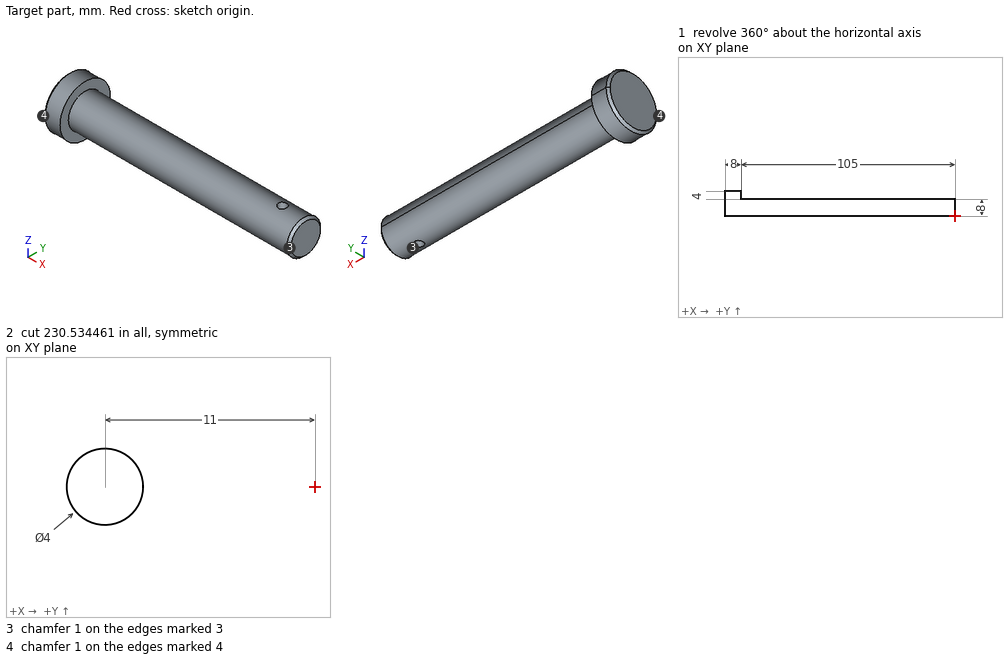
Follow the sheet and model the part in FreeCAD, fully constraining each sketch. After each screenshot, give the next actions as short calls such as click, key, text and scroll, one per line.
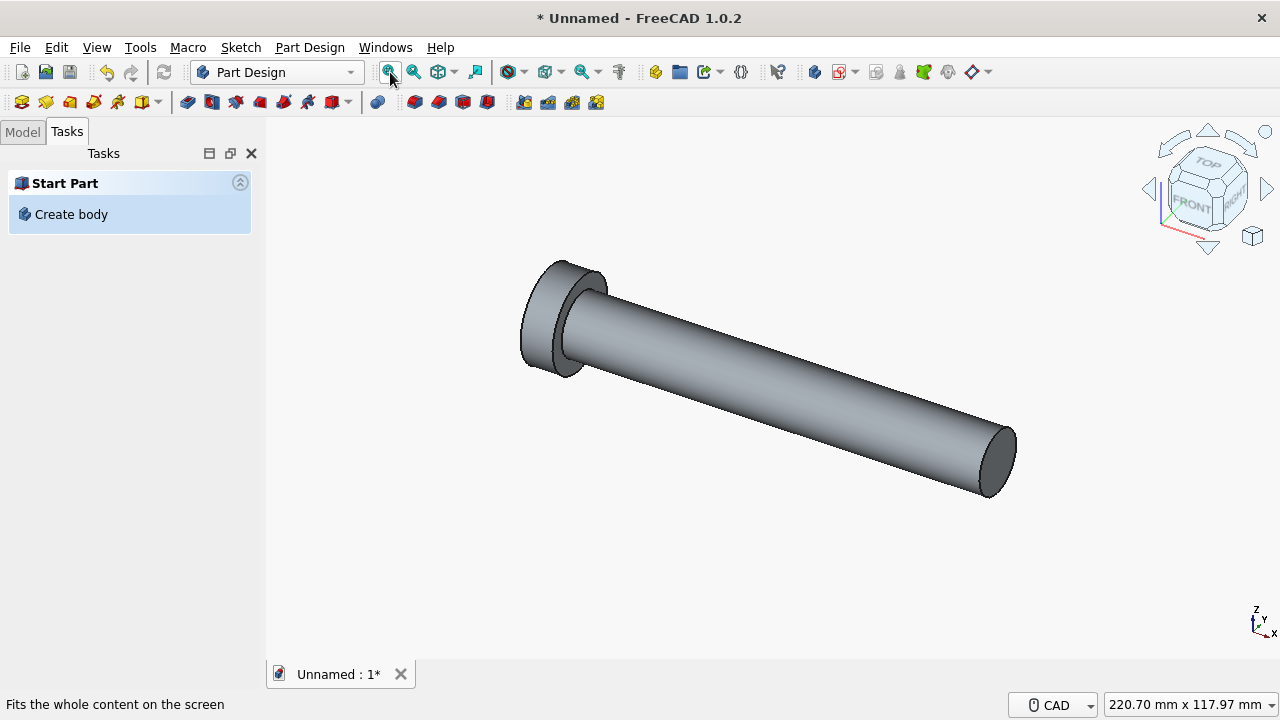
click(840, 72)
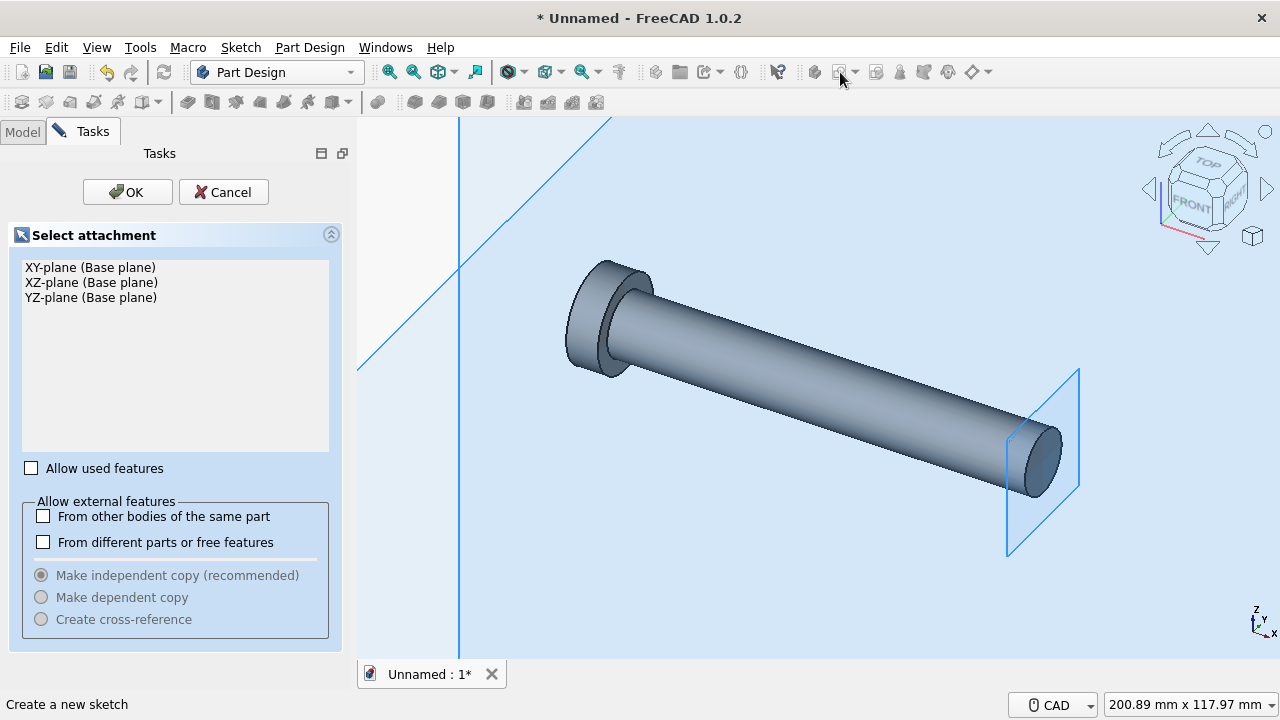
click(82, 268)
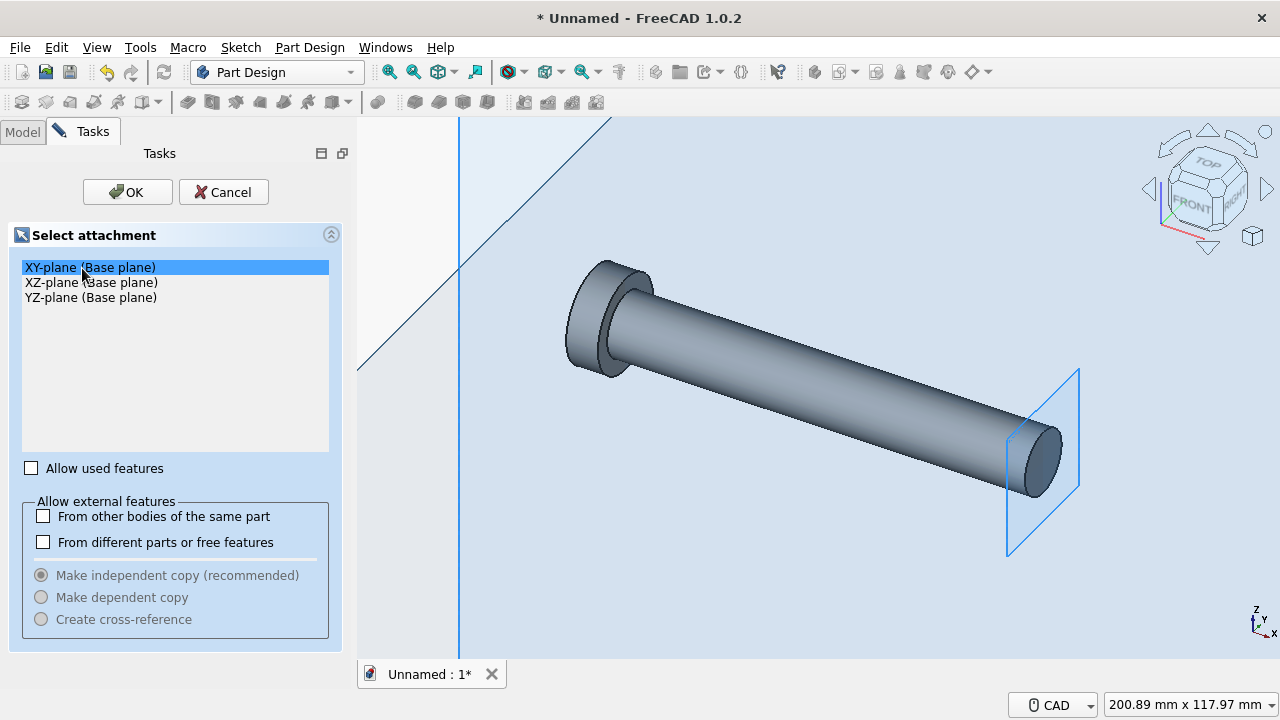
click(128, 192)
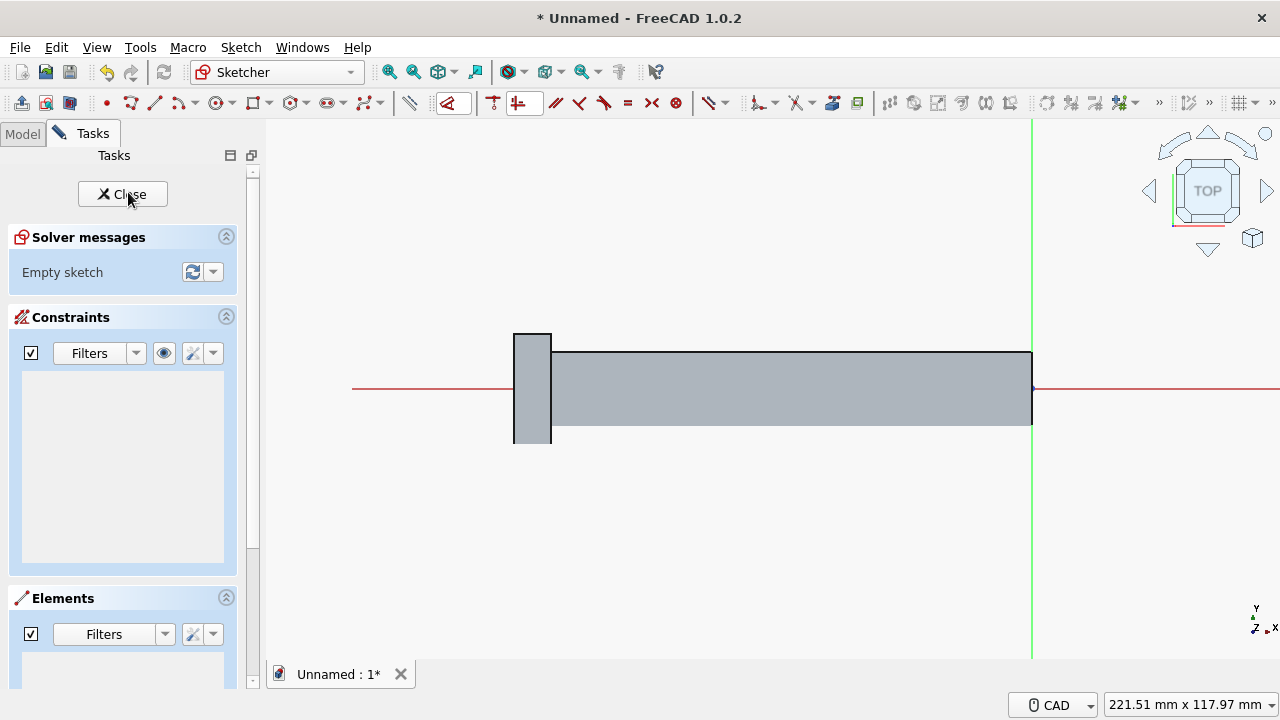
click(70, 104)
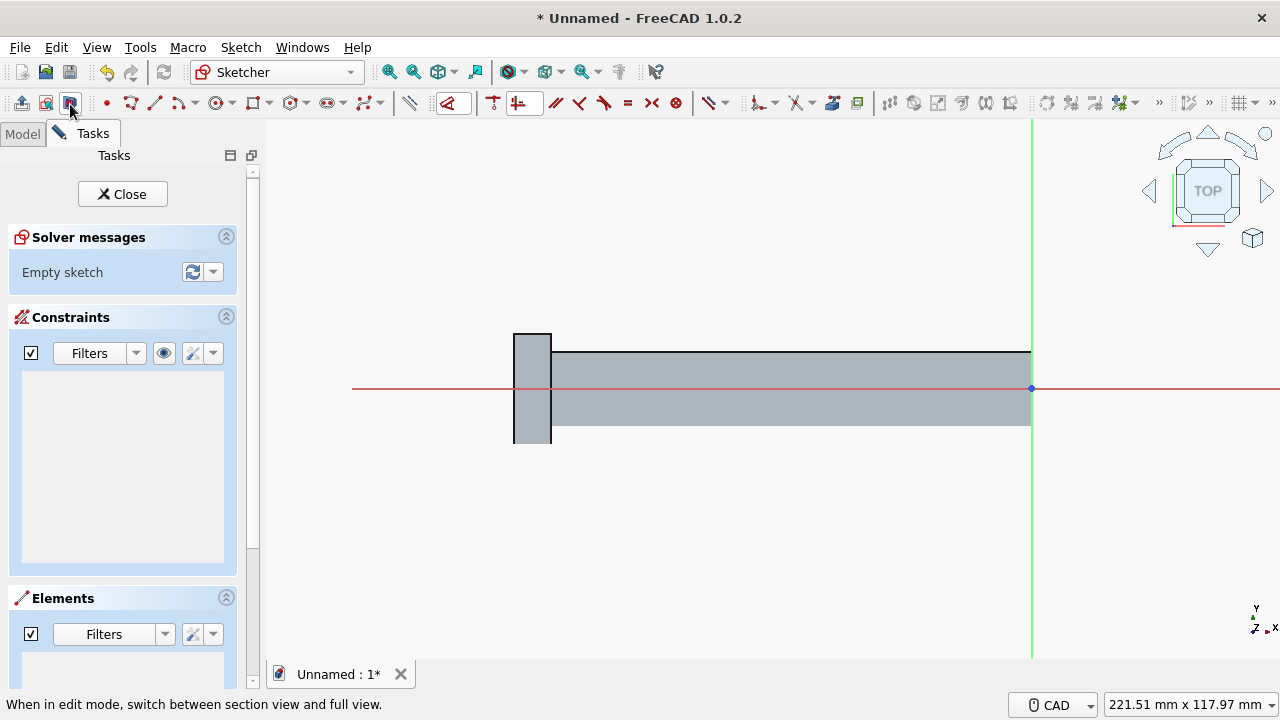
scroll(996, 389, up, 15)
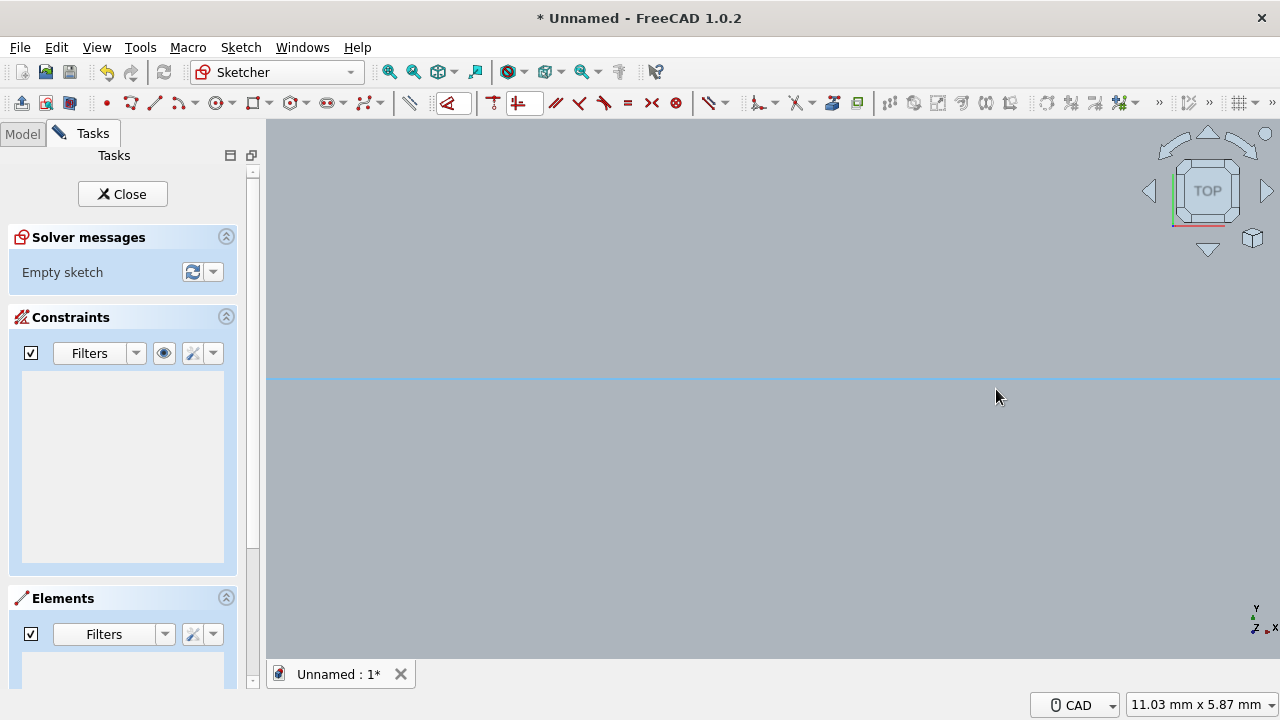
click(216, 104)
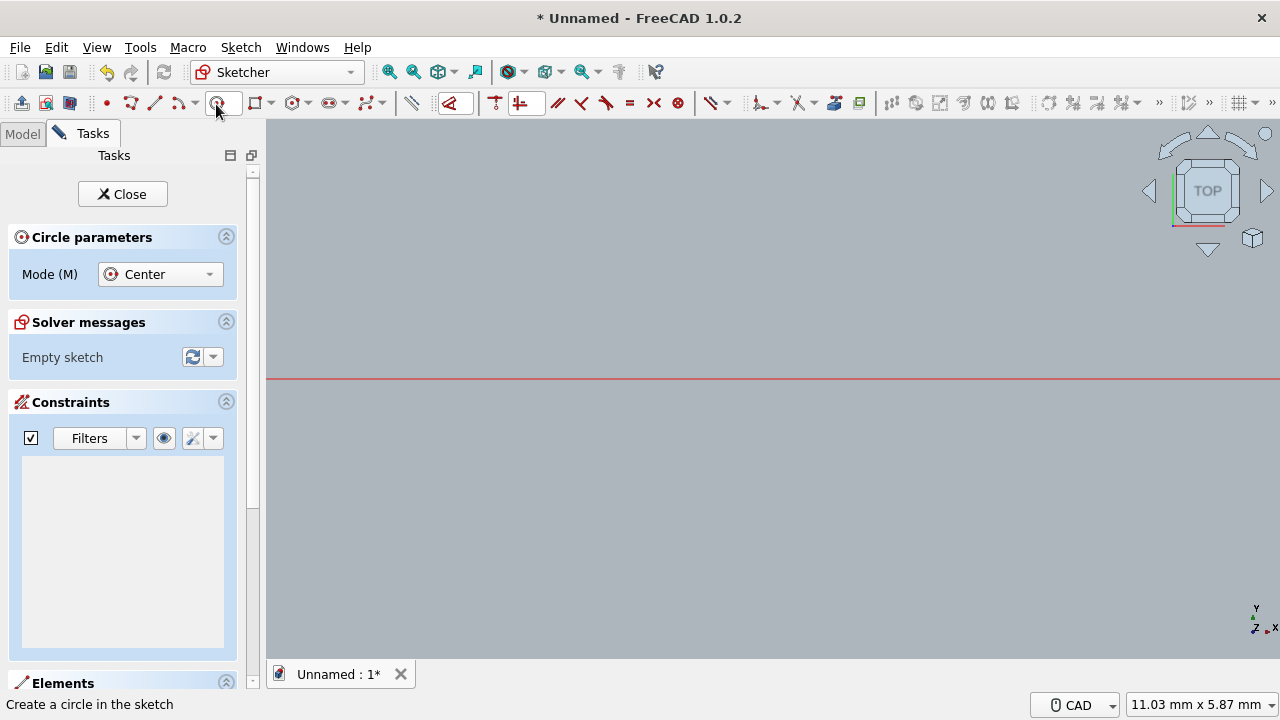
click(687, 379)
move(817, 249)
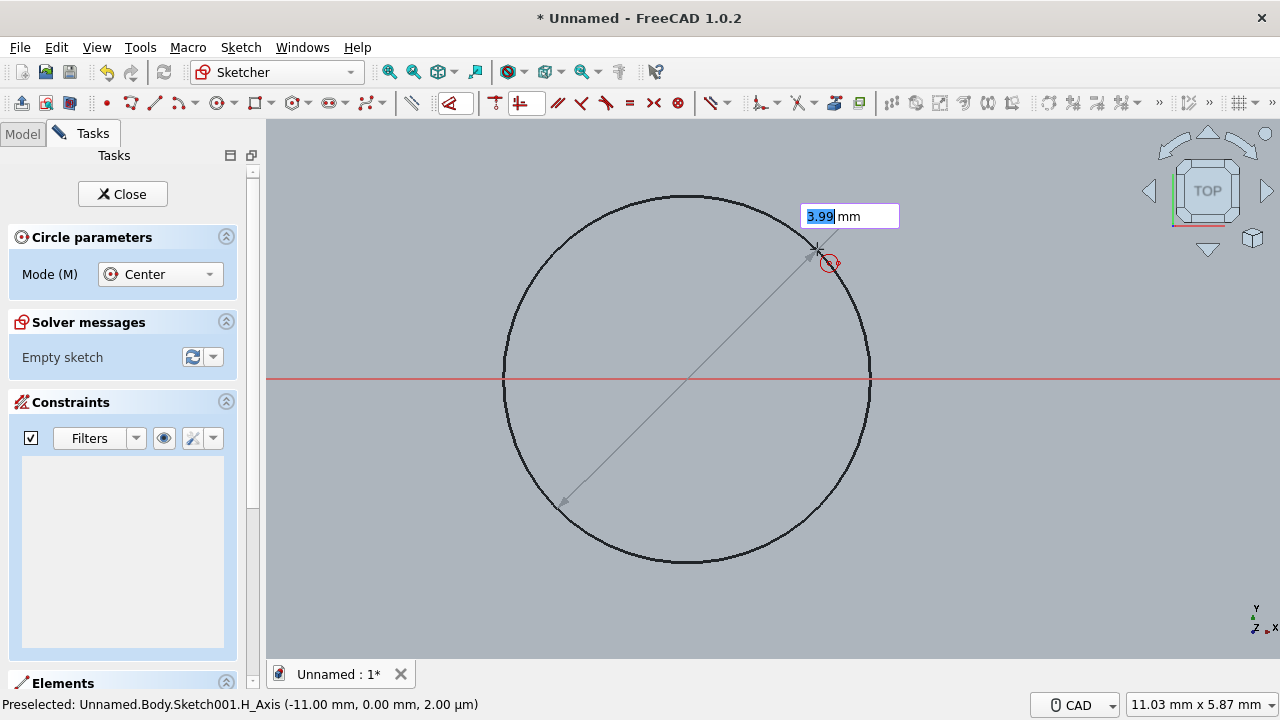
text(4)
key(Return)
key(Escape)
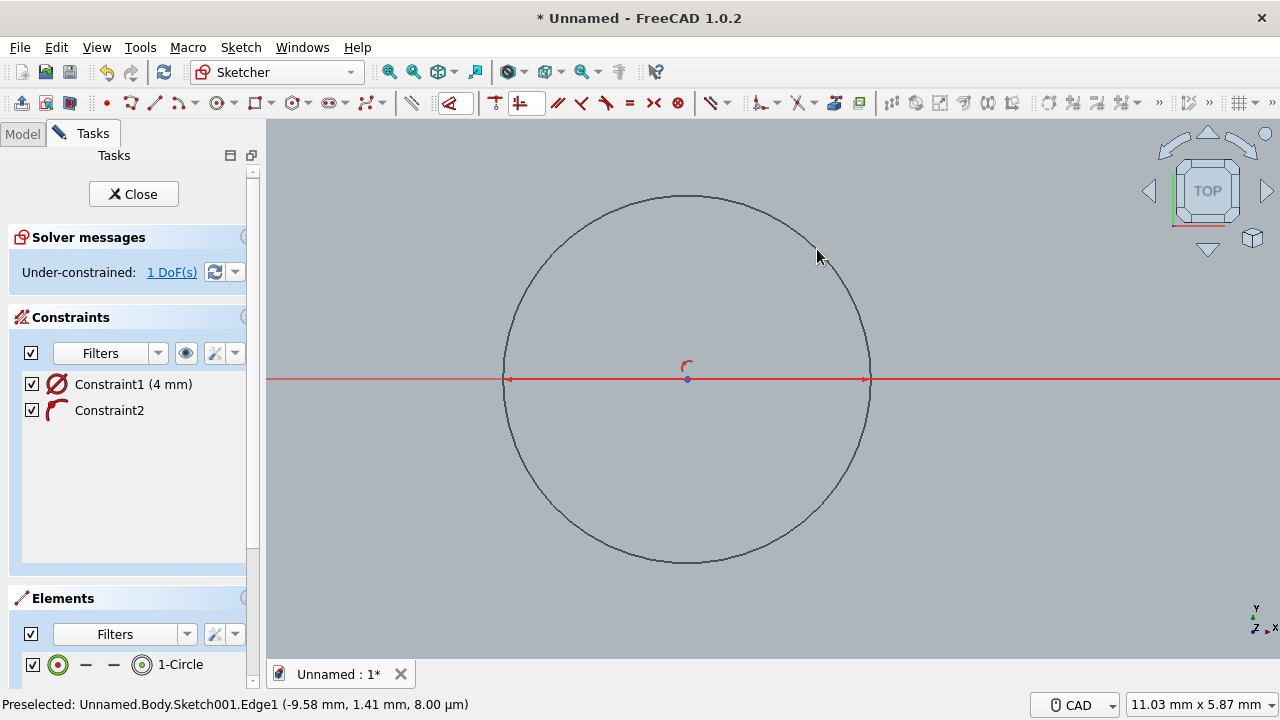
click(687, 379)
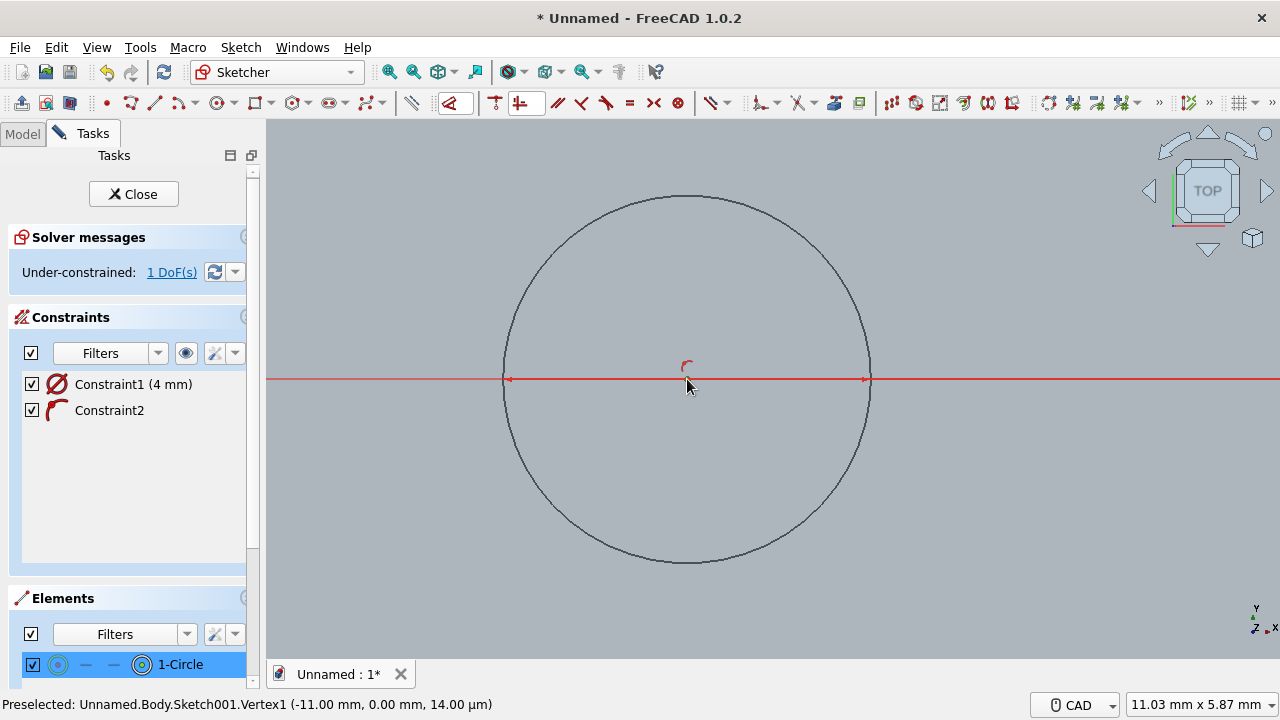
click(468, 104)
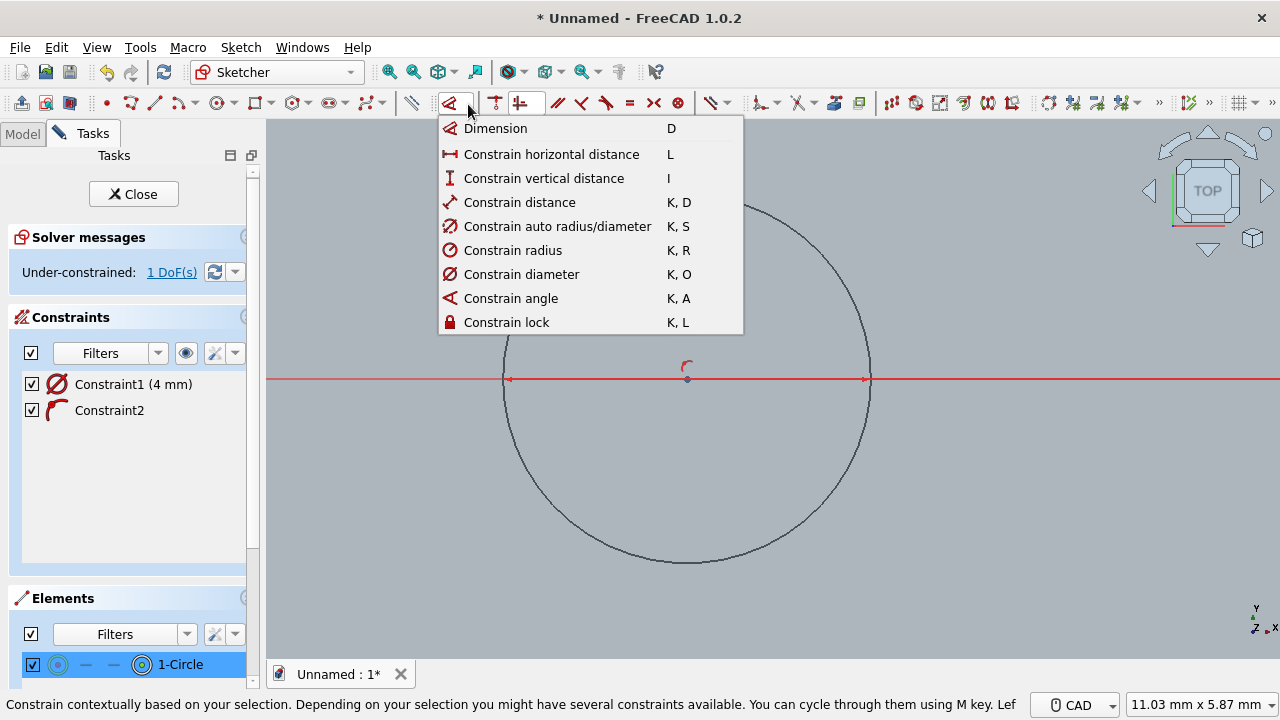
click(591, 154)